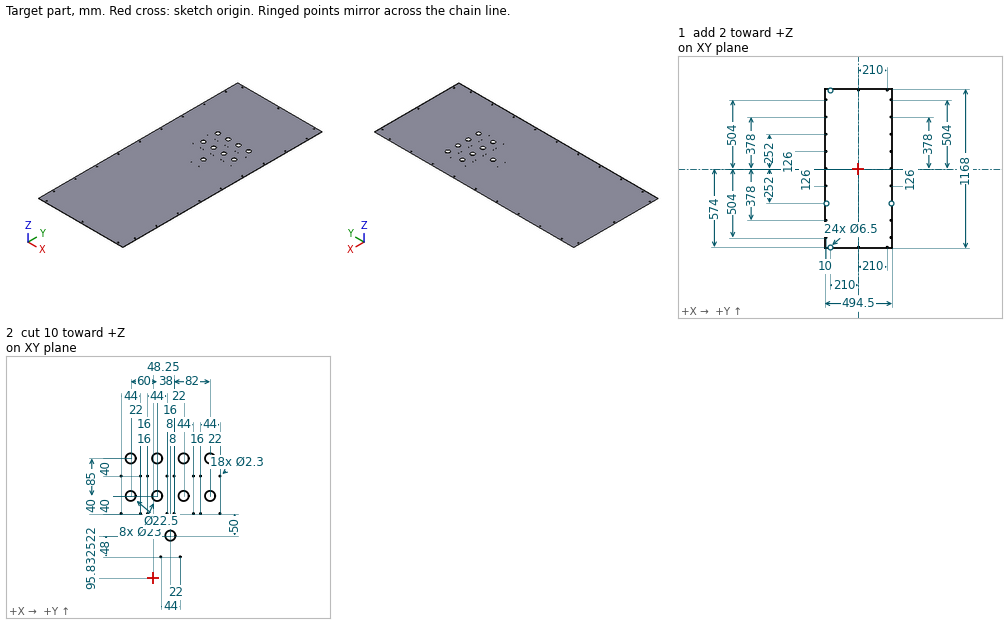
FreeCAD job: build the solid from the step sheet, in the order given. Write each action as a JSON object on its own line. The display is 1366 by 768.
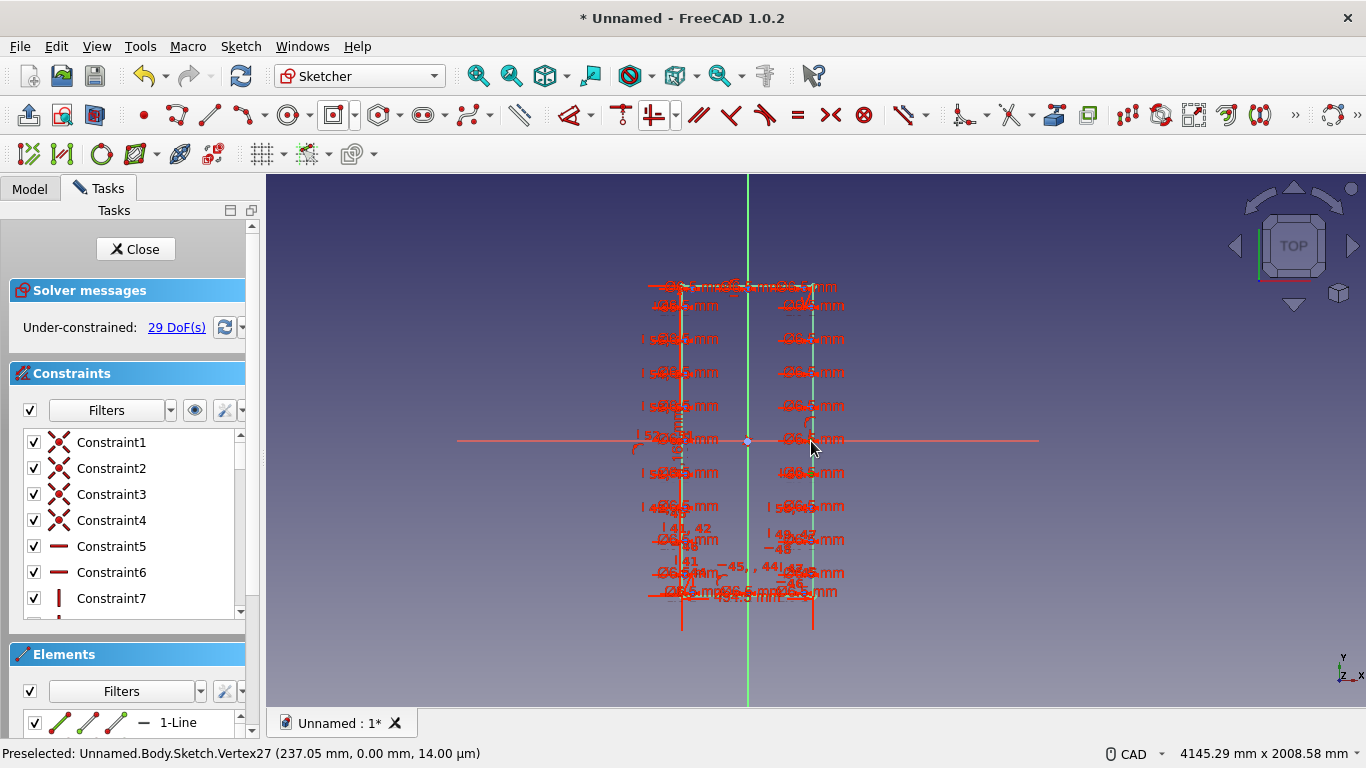
{"action": "left_click", "coordinate": [676, 116]}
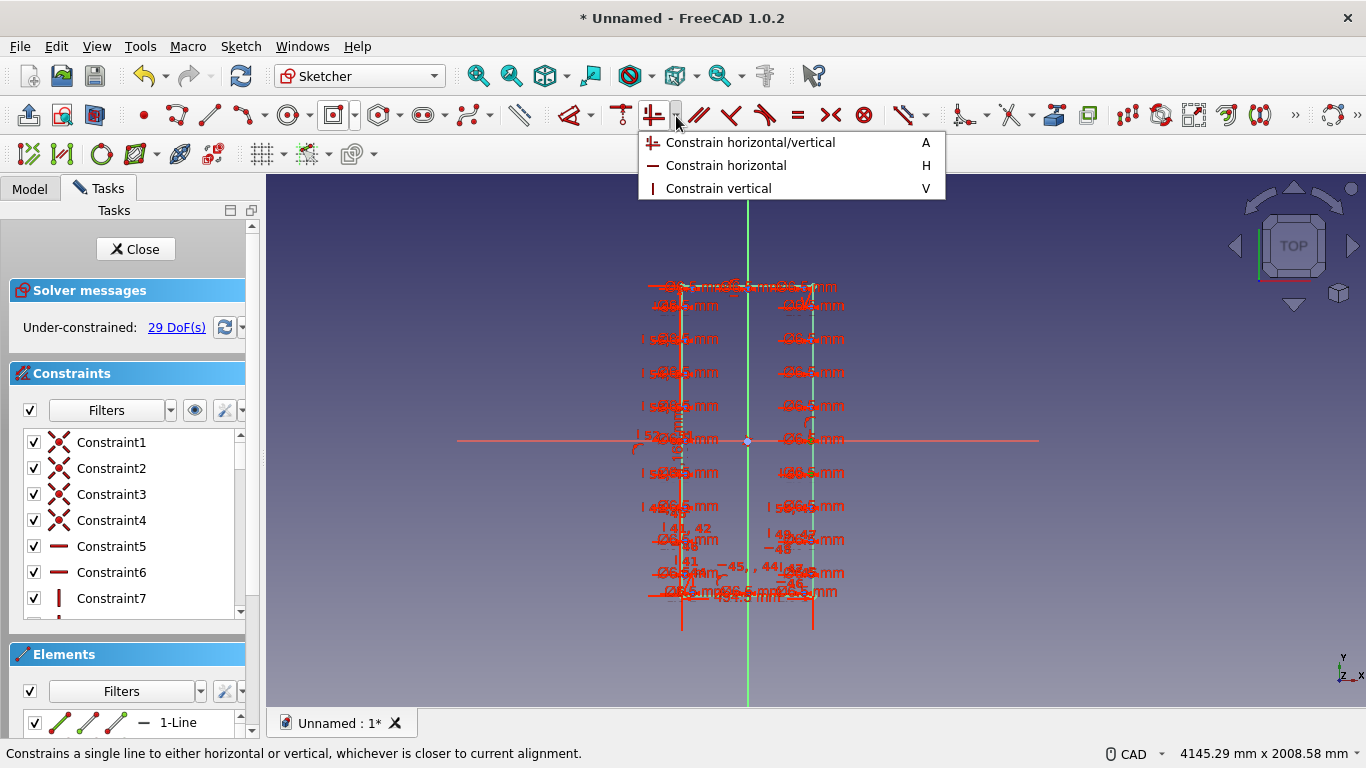
{"action": "left_click", "coordinate": [792, 188]}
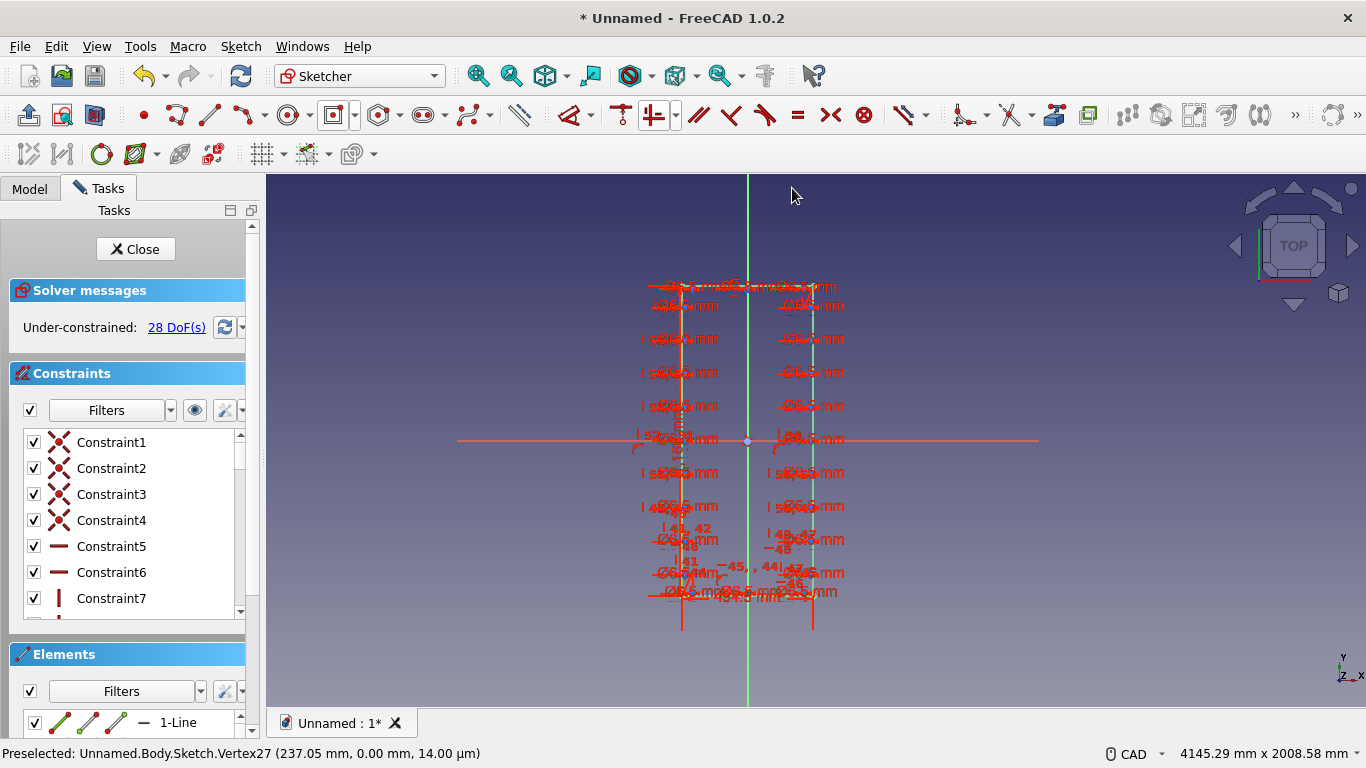
{"action": "left_click", "coordinate": [811, 441]}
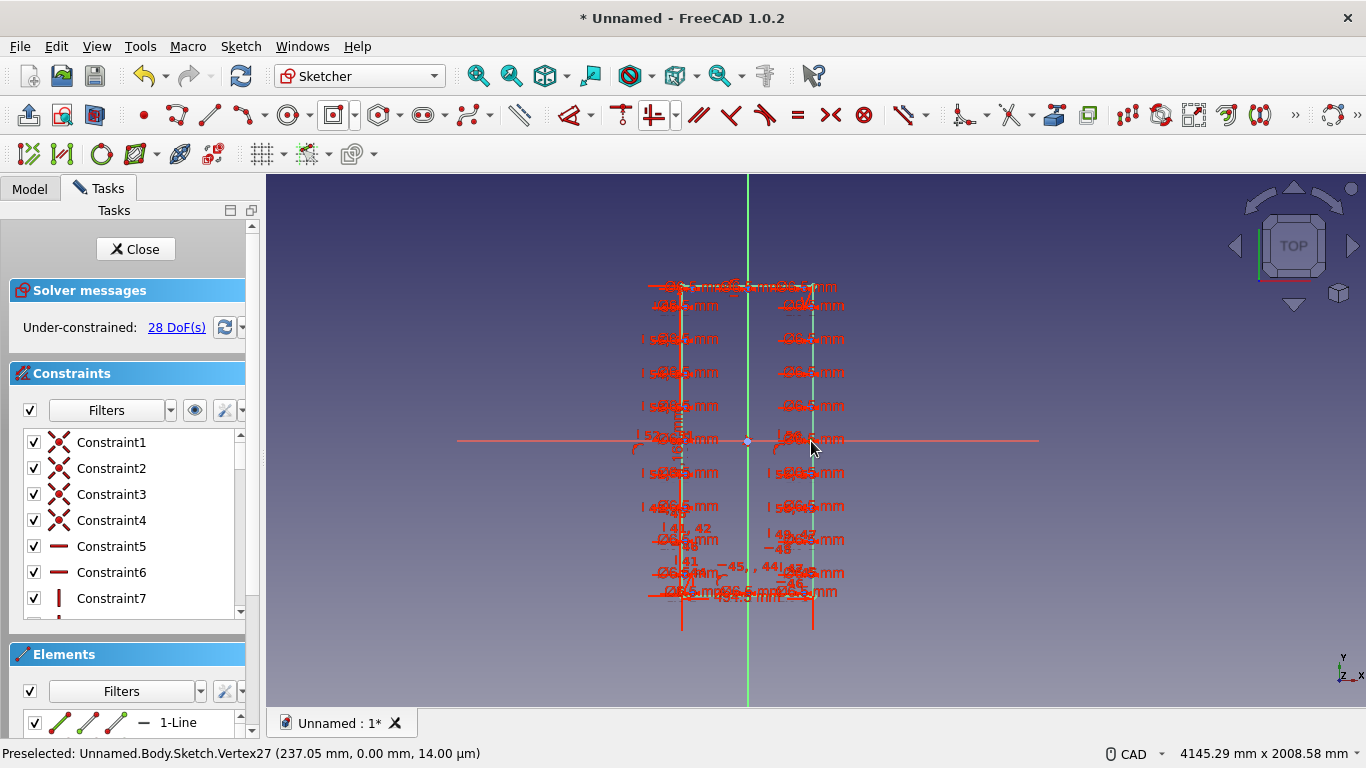
{"action": "left_click", "coordinate": [811, 408]}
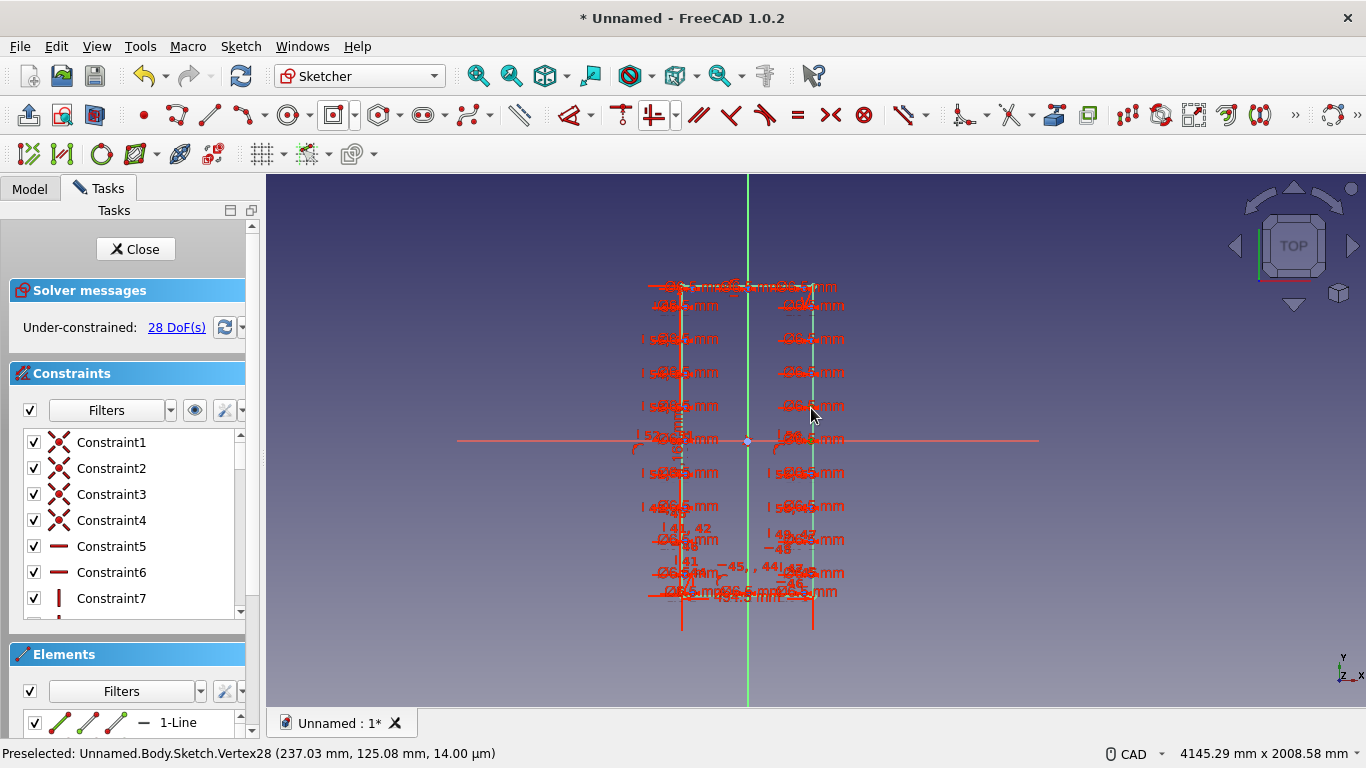
{"action": "left_click", "coordinate": [676, 116]}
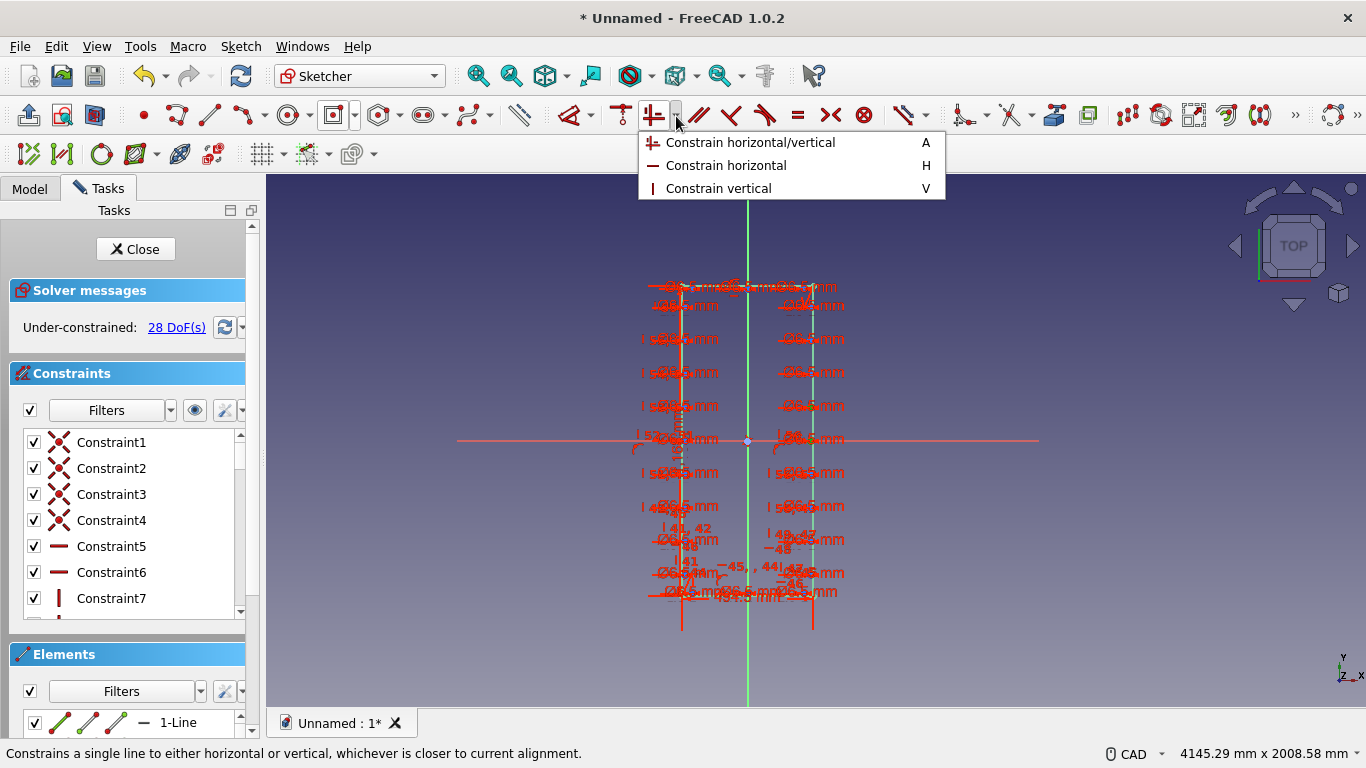
{"action": "left_click", "coordinate": [792, 188]}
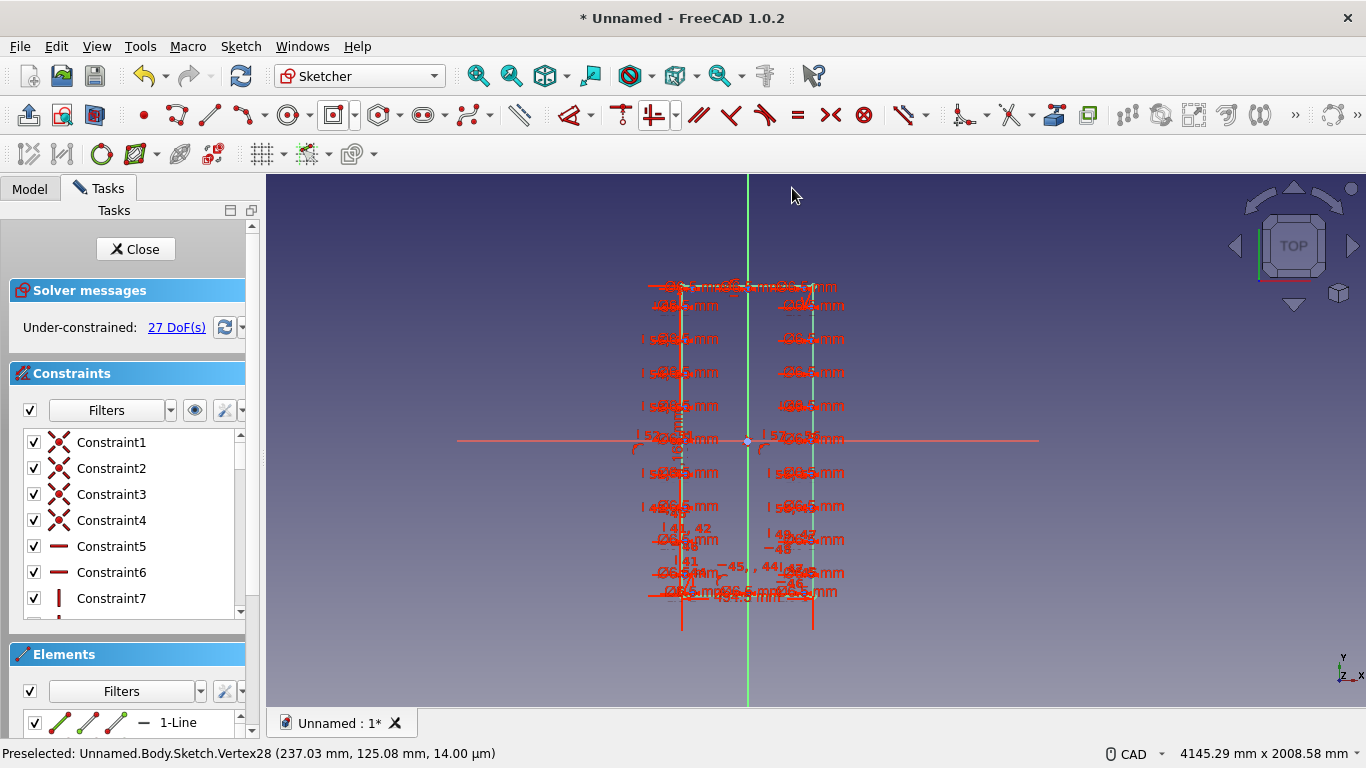
{"action": "left_click", "coordinate": [685, 408]}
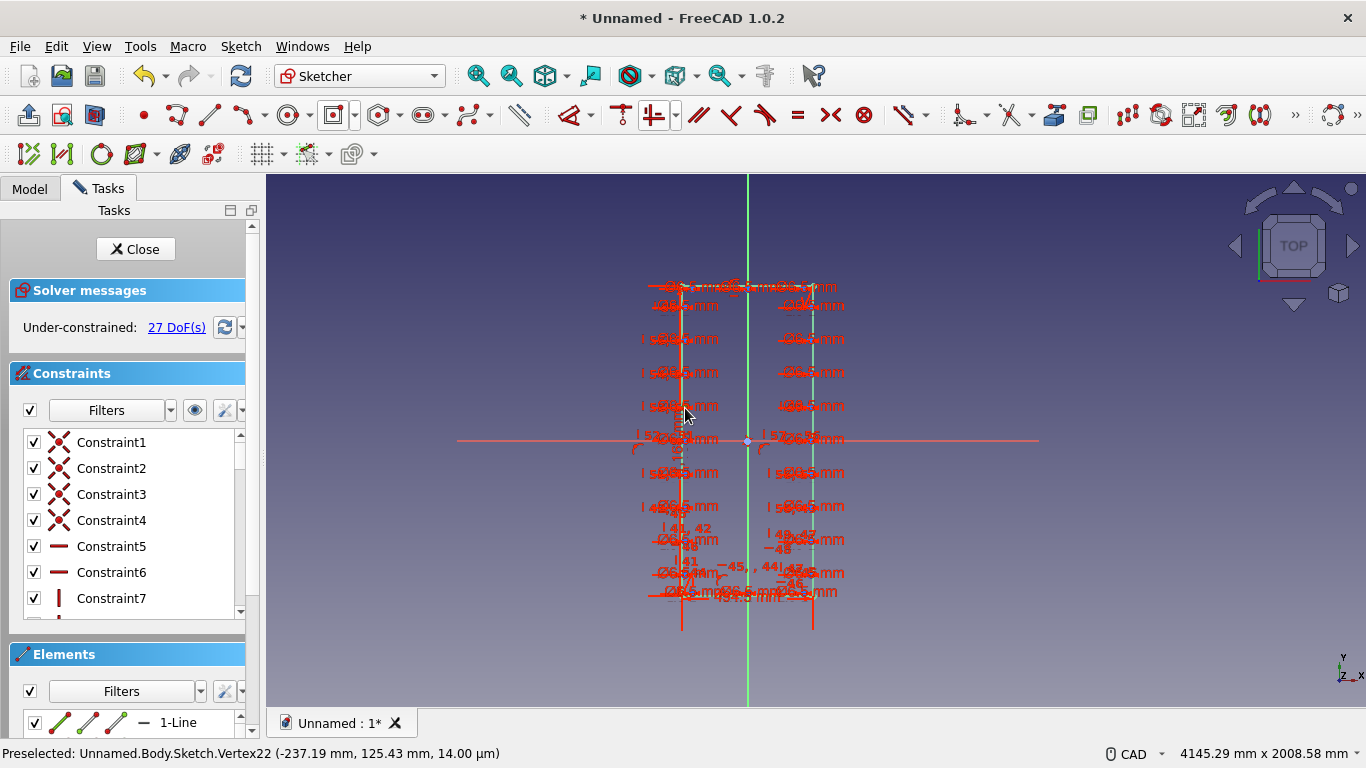
{"action": "left_click", "coordinate": [811, 408]}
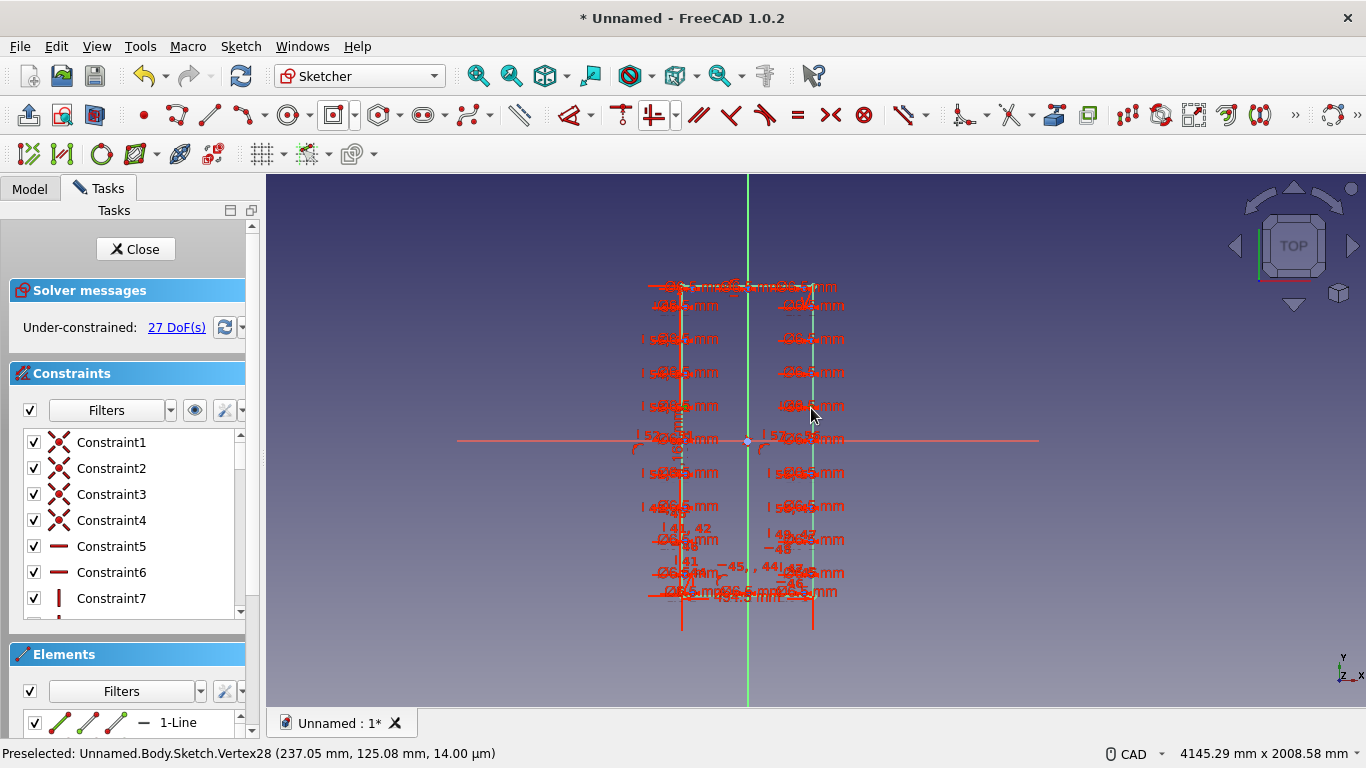
{"action": "left_click", "coordinate": [676, 116]}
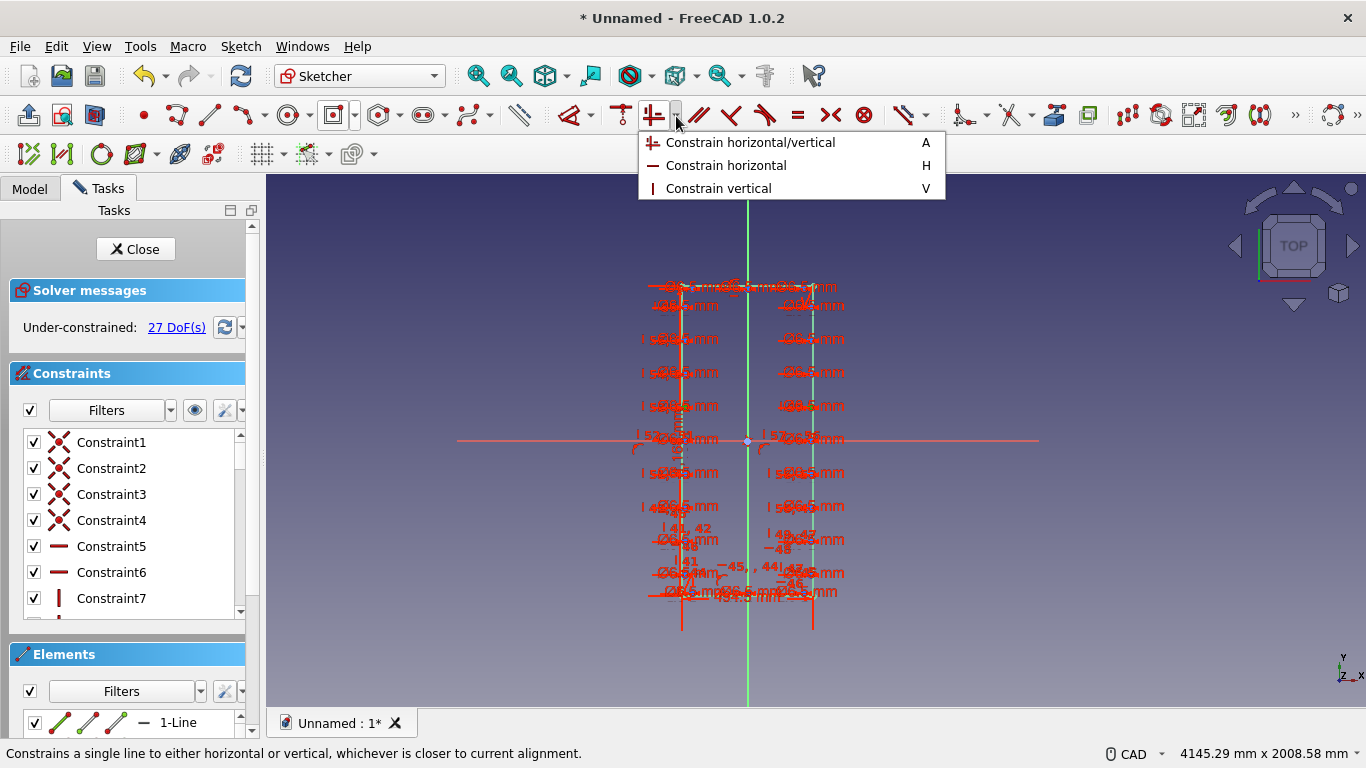
{"action": "left_click", "coordinate": [792, 166]}